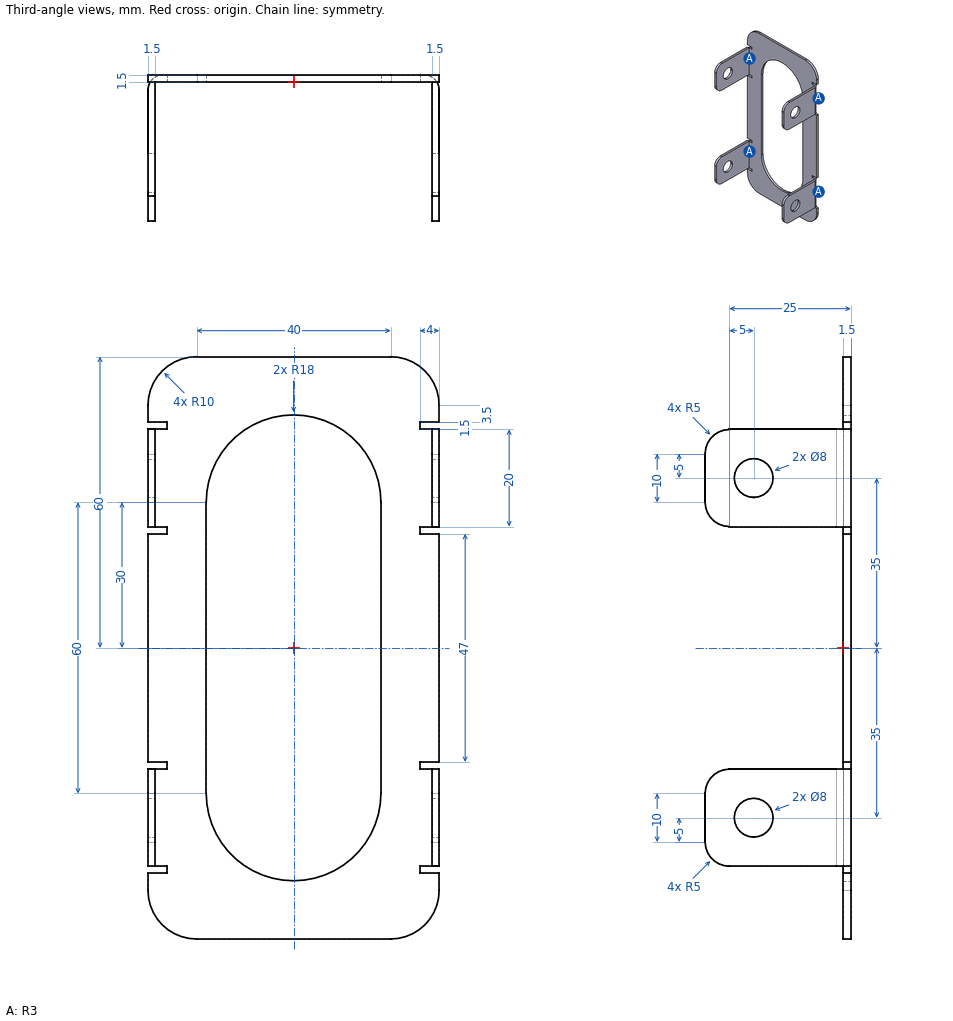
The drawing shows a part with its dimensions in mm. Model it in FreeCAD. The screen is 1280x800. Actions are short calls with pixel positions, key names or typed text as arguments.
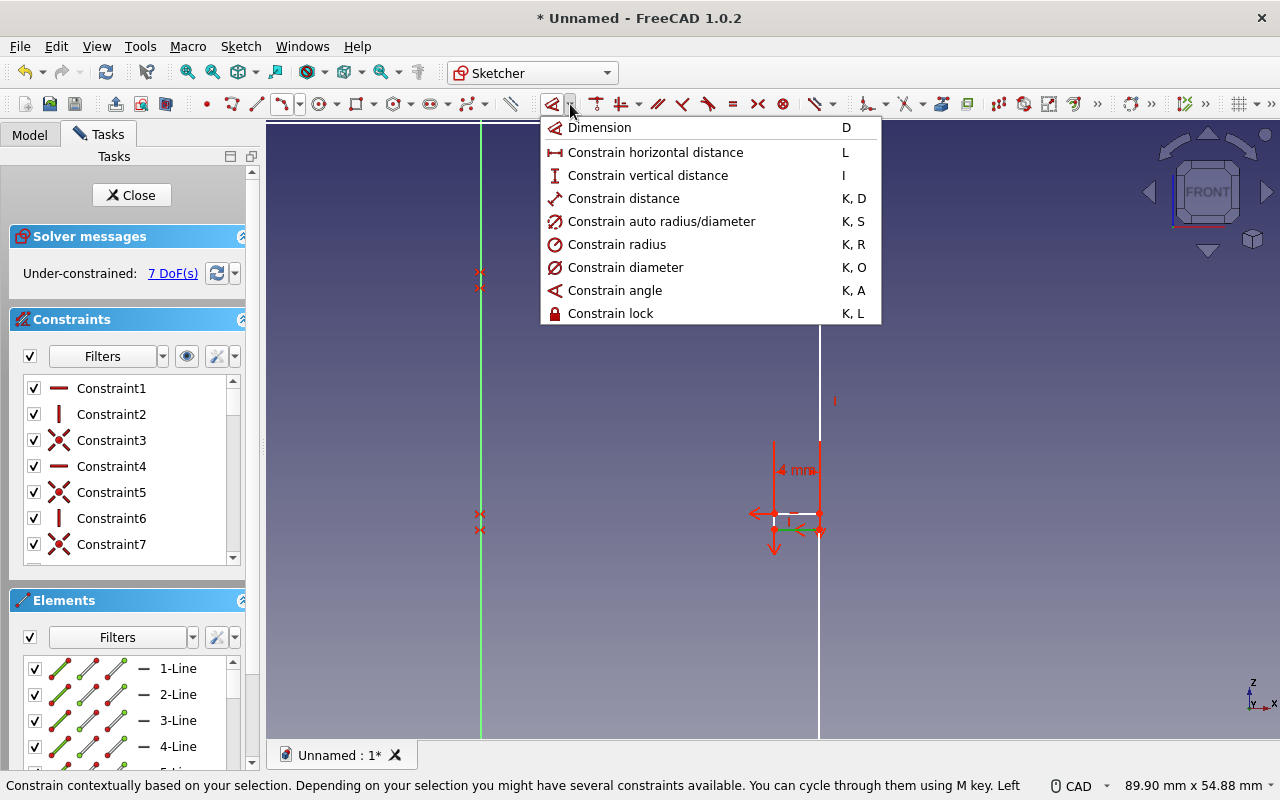
click(711, 152)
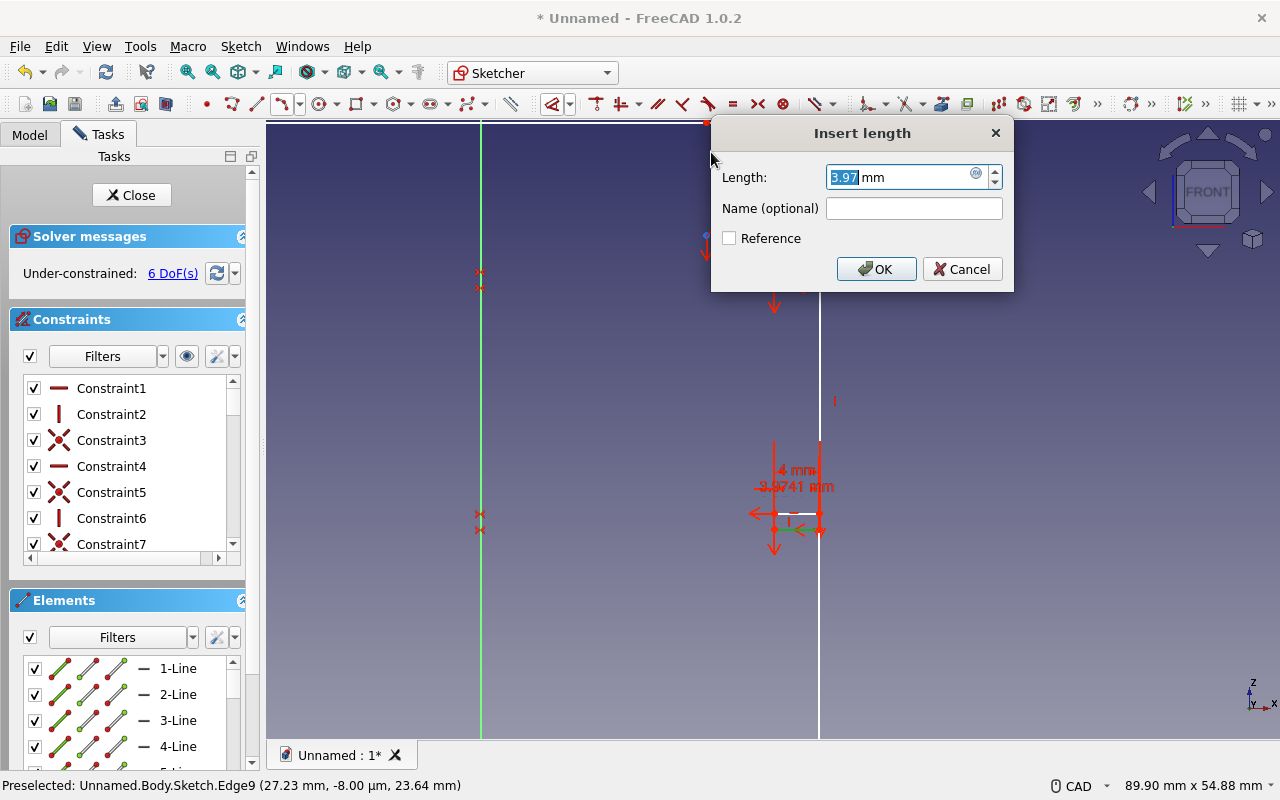
text(4)
key(Return)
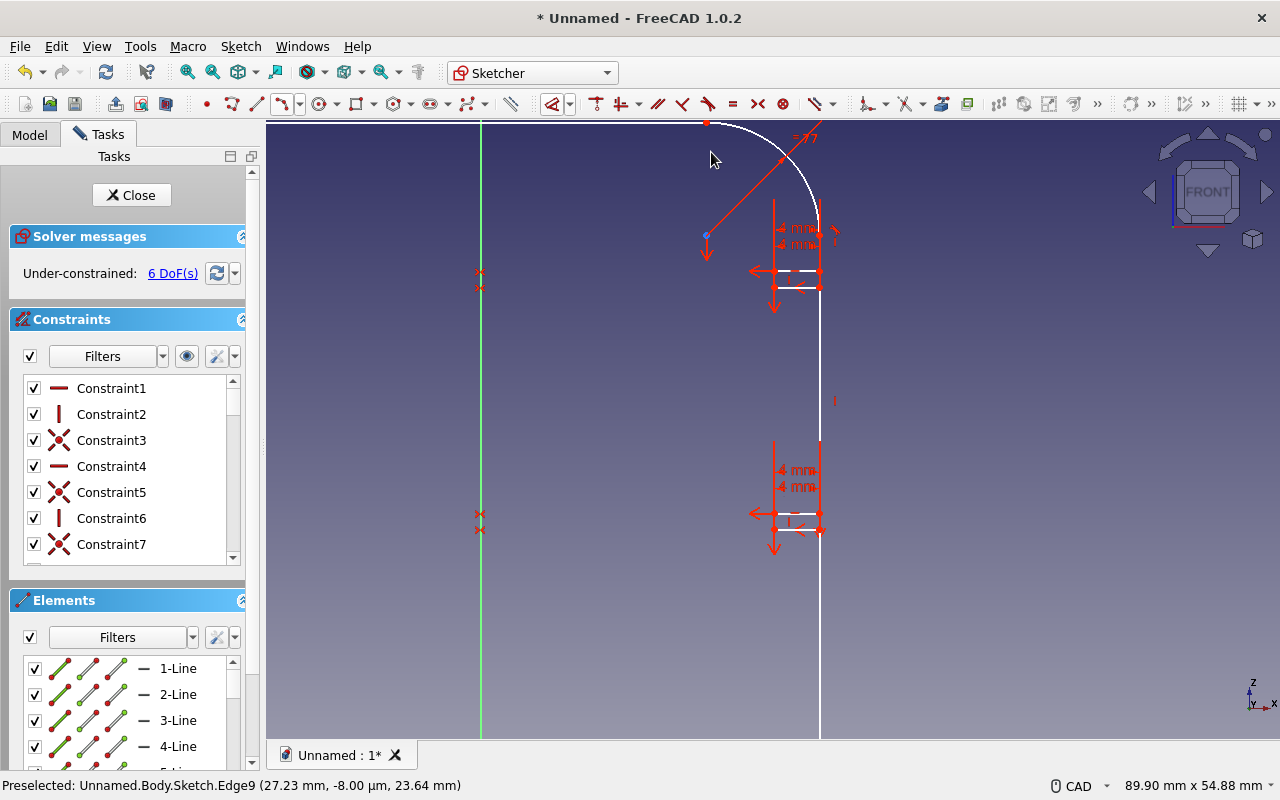
scroll(801, 271, down, 6)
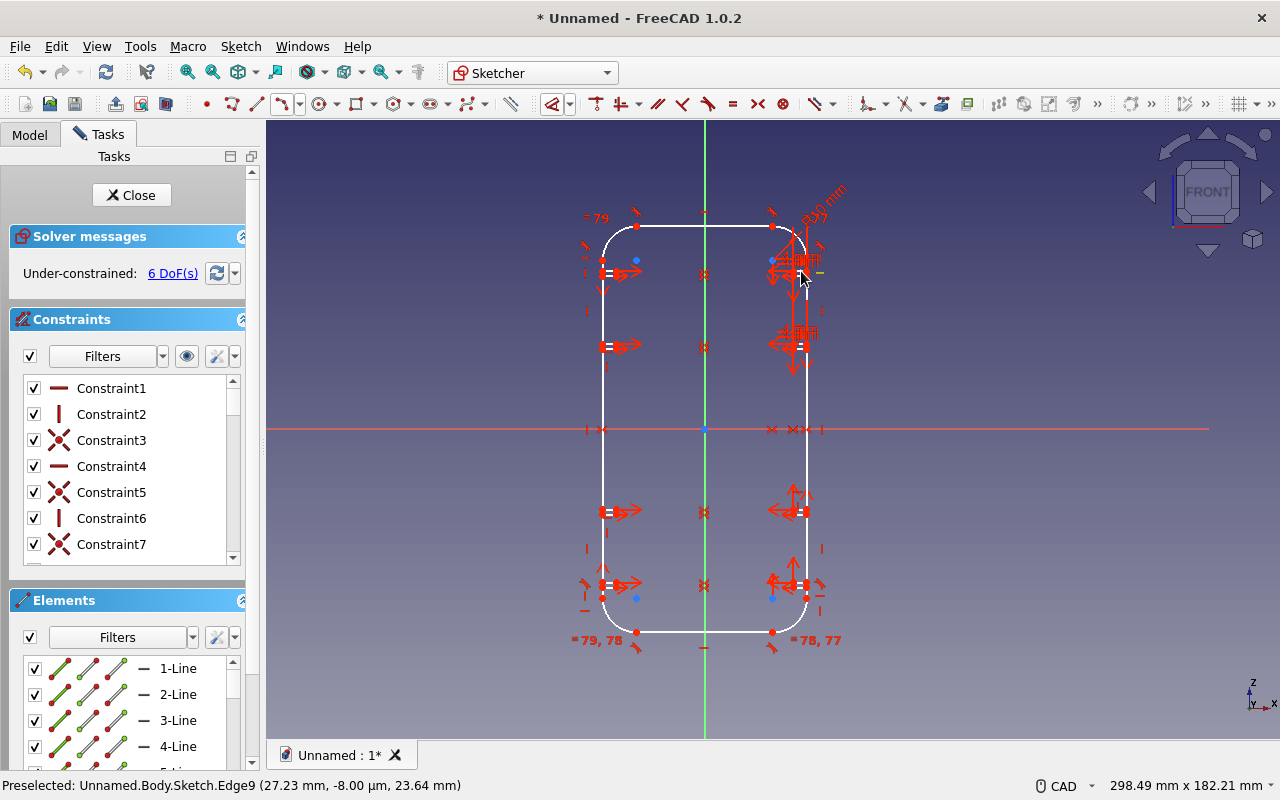
click(678, 226)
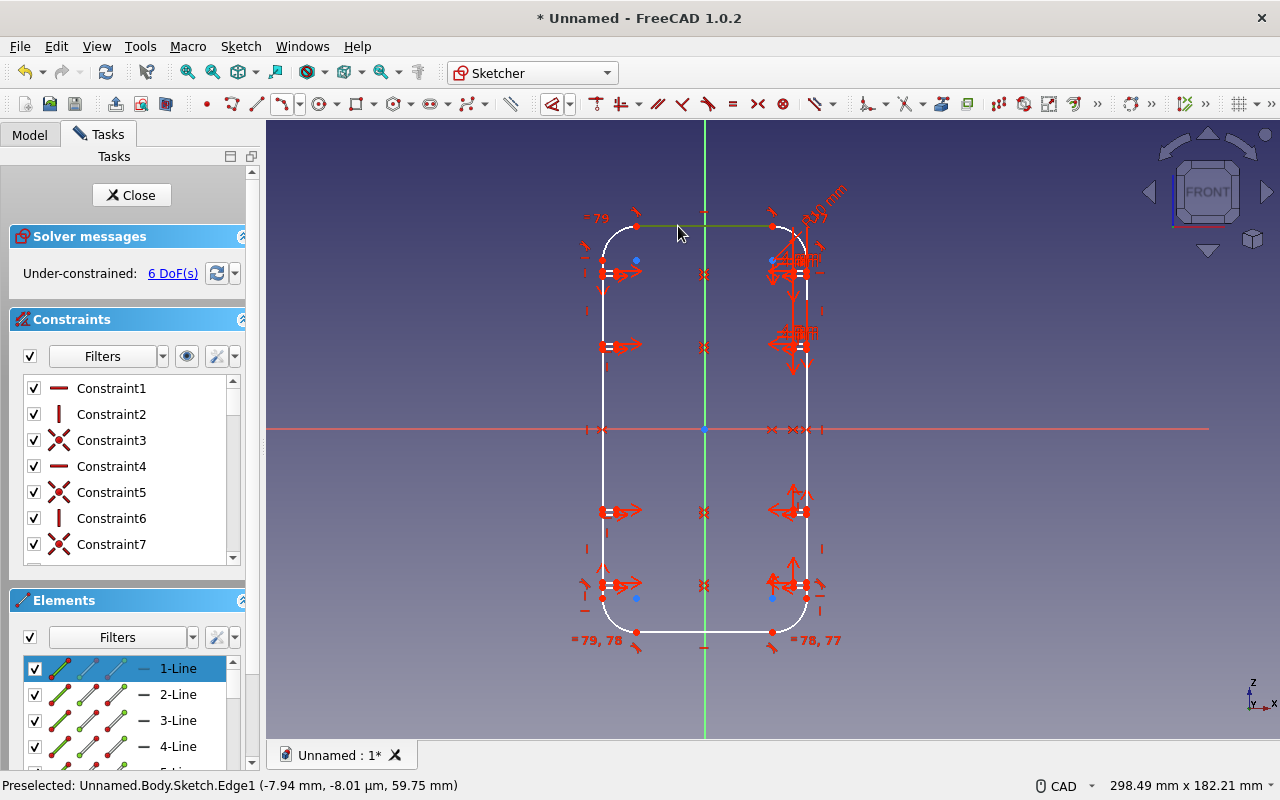
click(570, 104)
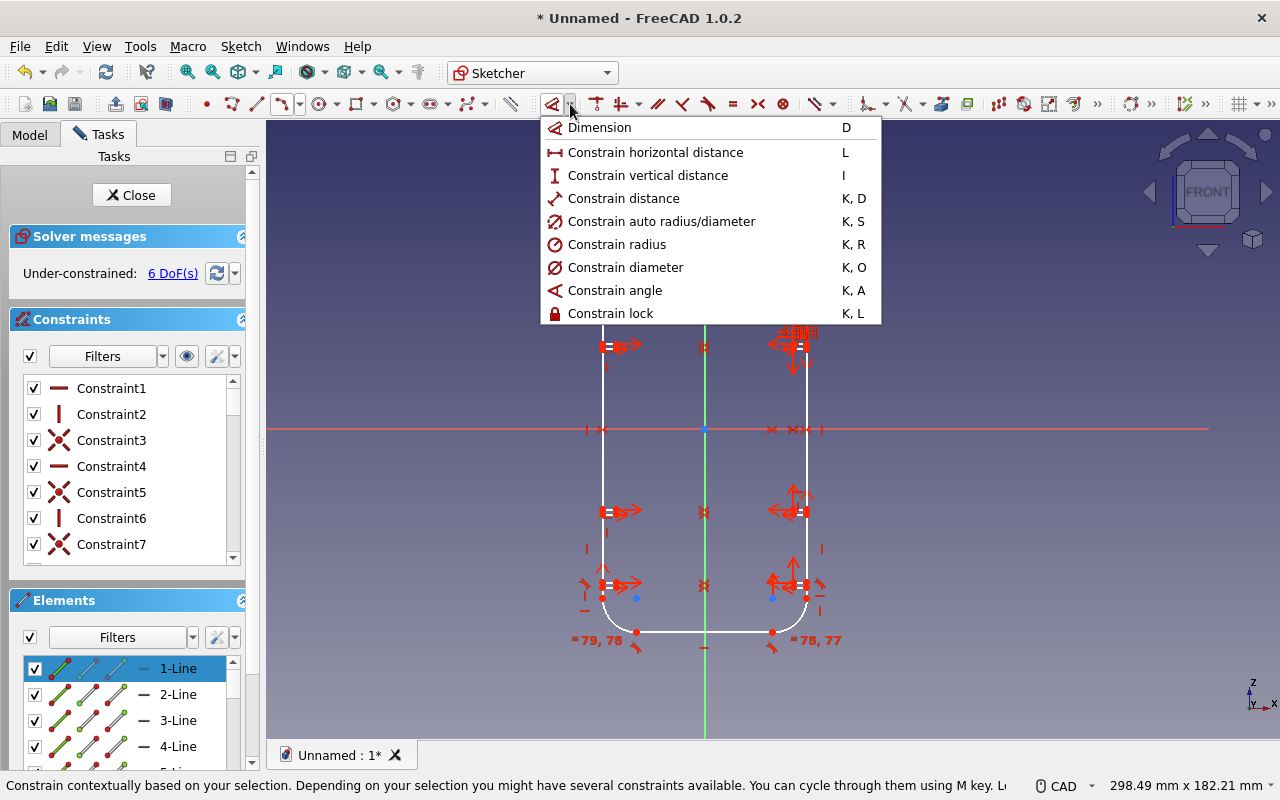
click(711, 152)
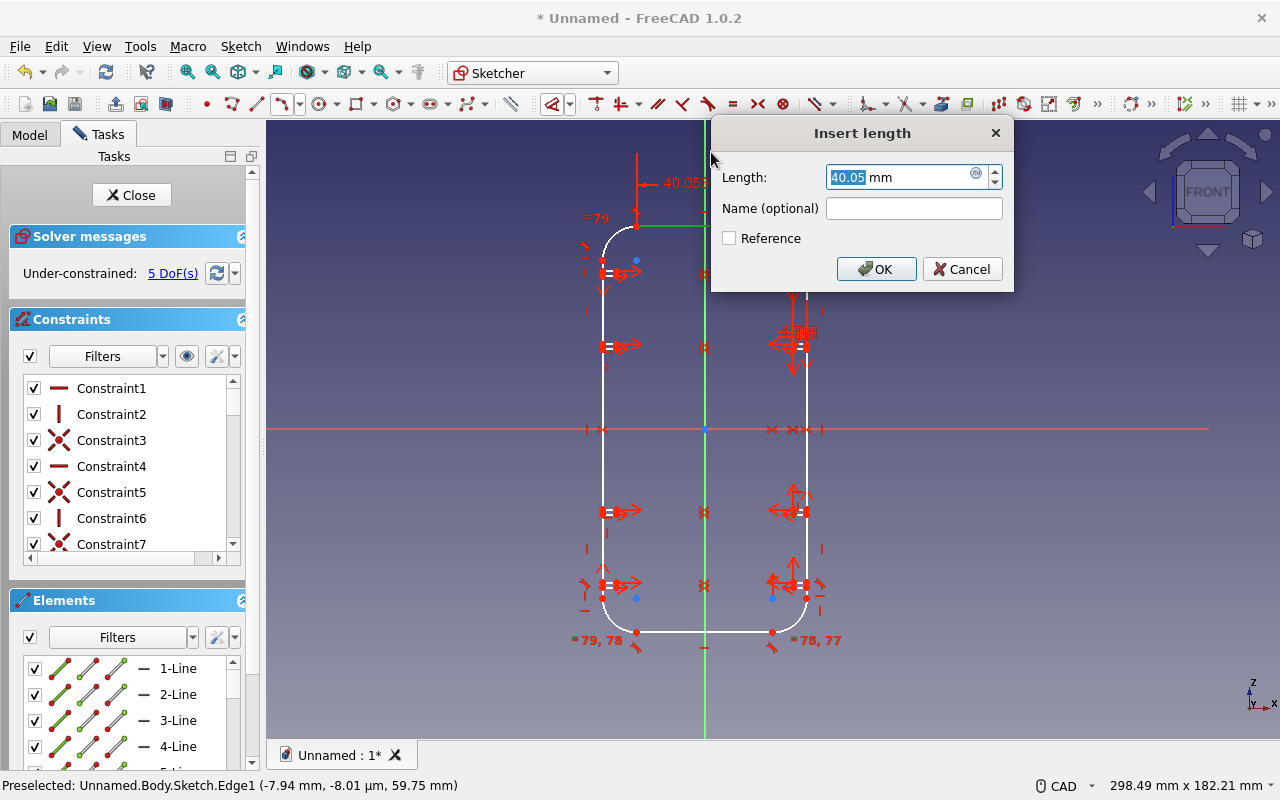
text(40)
key(Return)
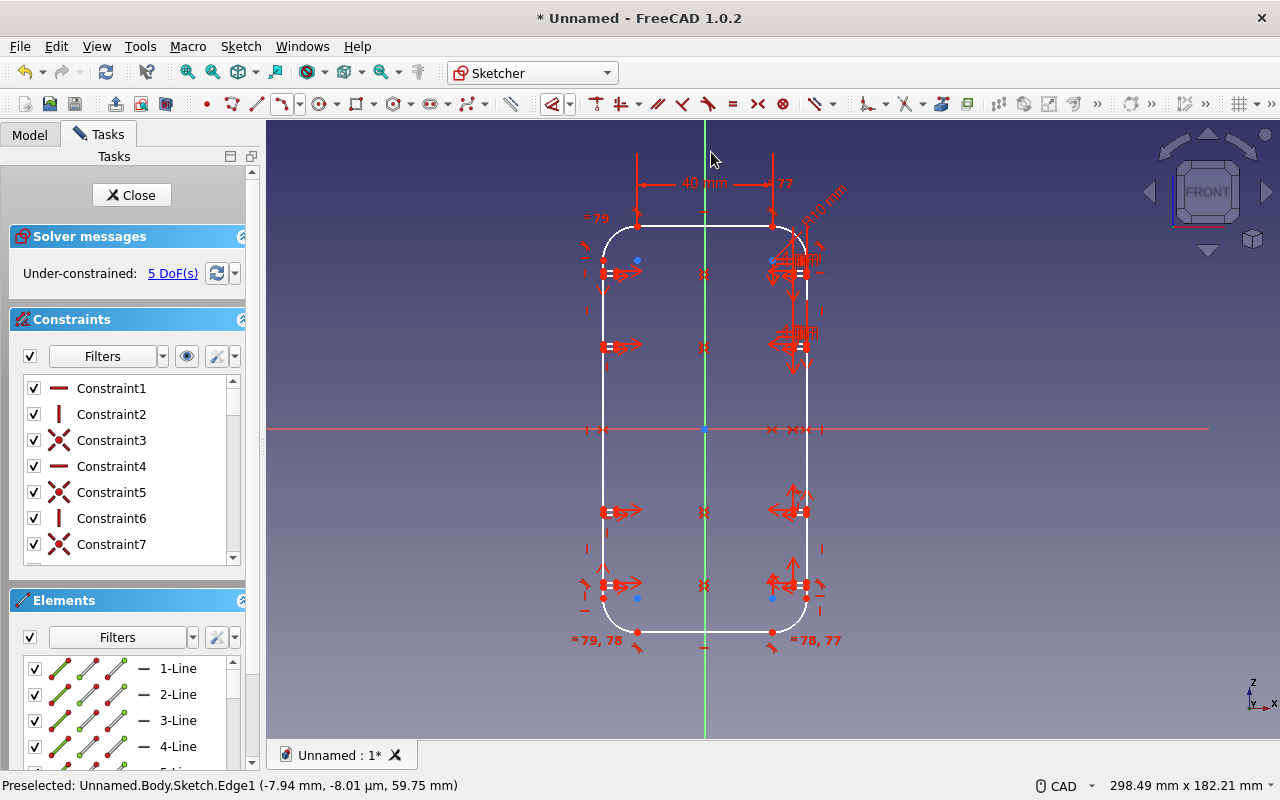
click(807, 297)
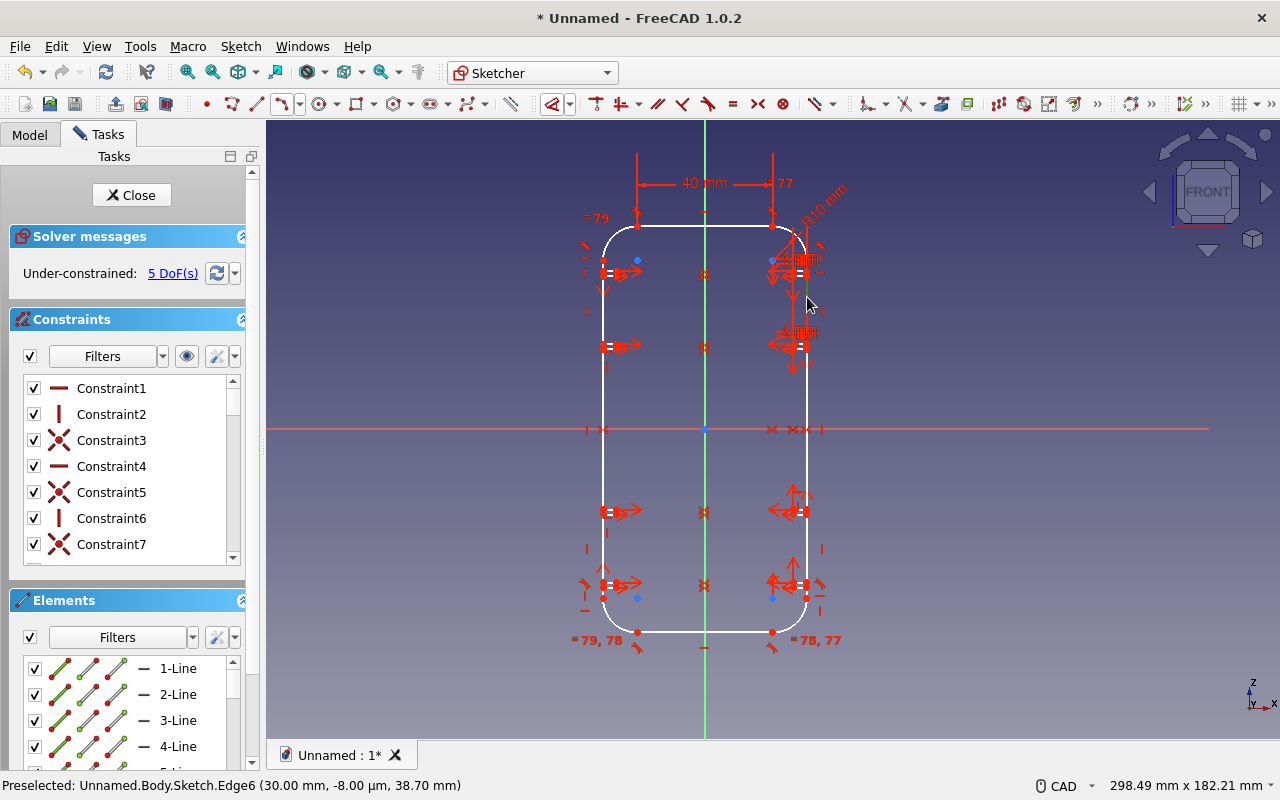
key(i)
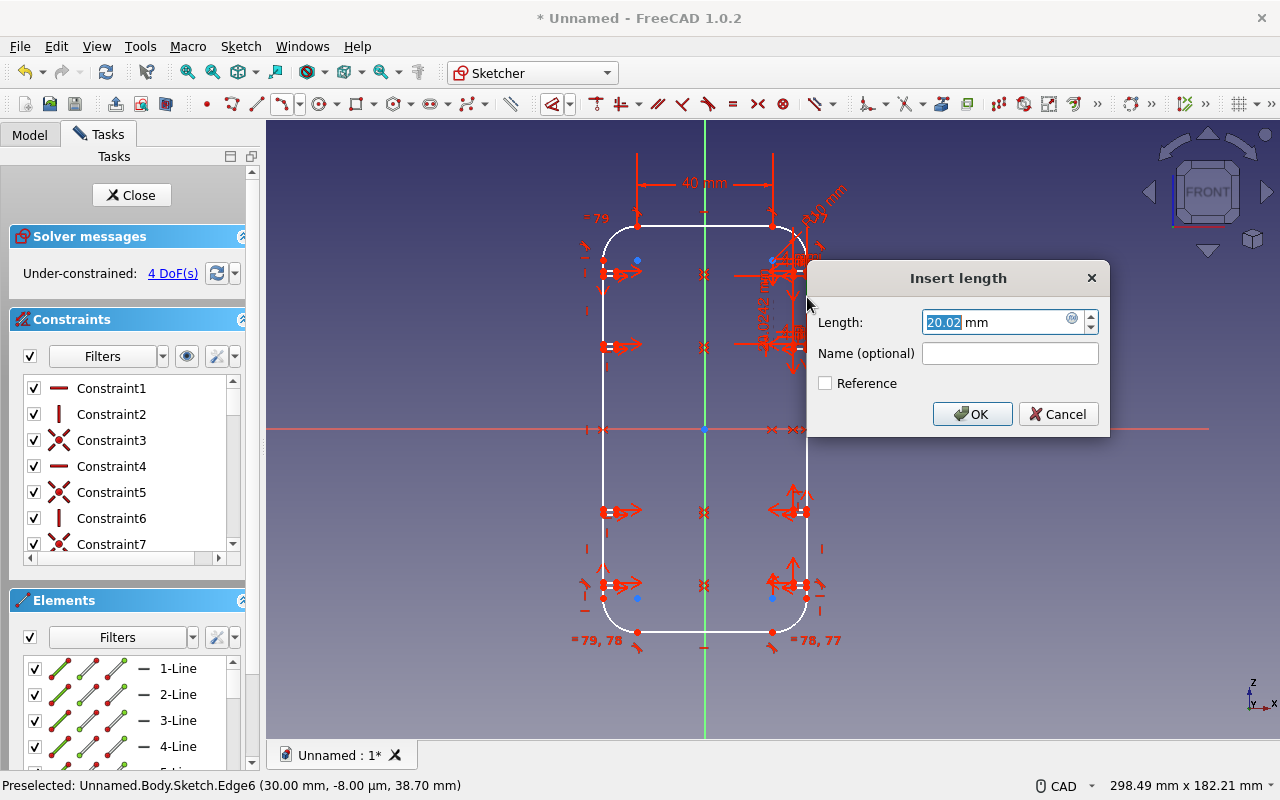
text(20)
key(Return)